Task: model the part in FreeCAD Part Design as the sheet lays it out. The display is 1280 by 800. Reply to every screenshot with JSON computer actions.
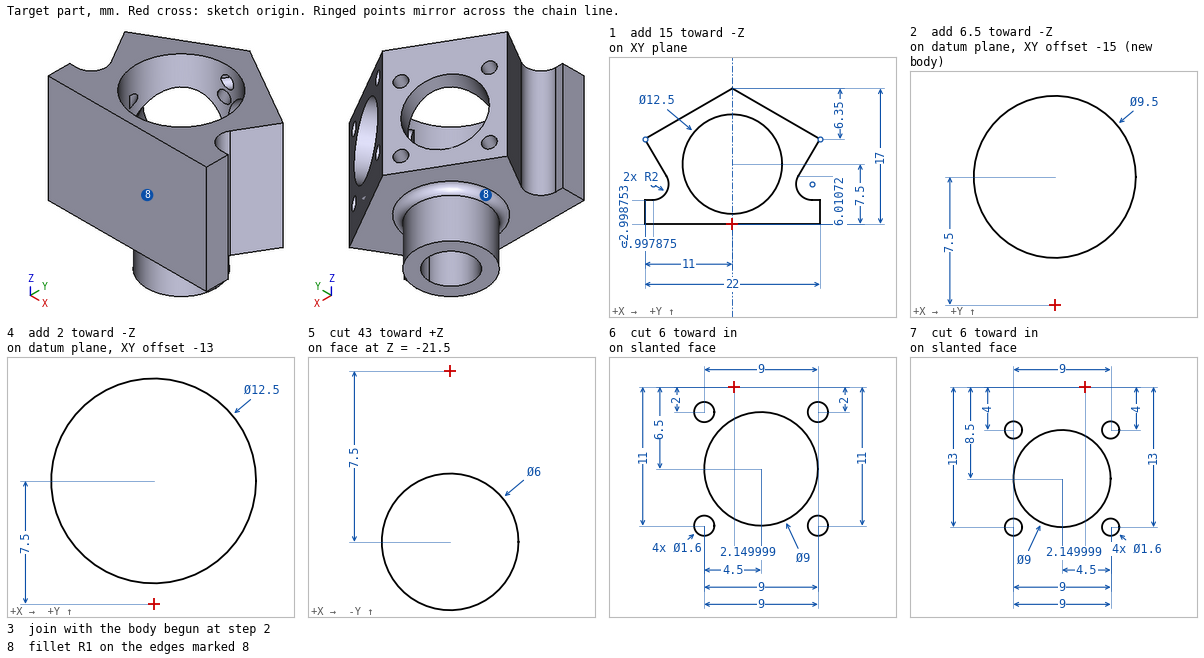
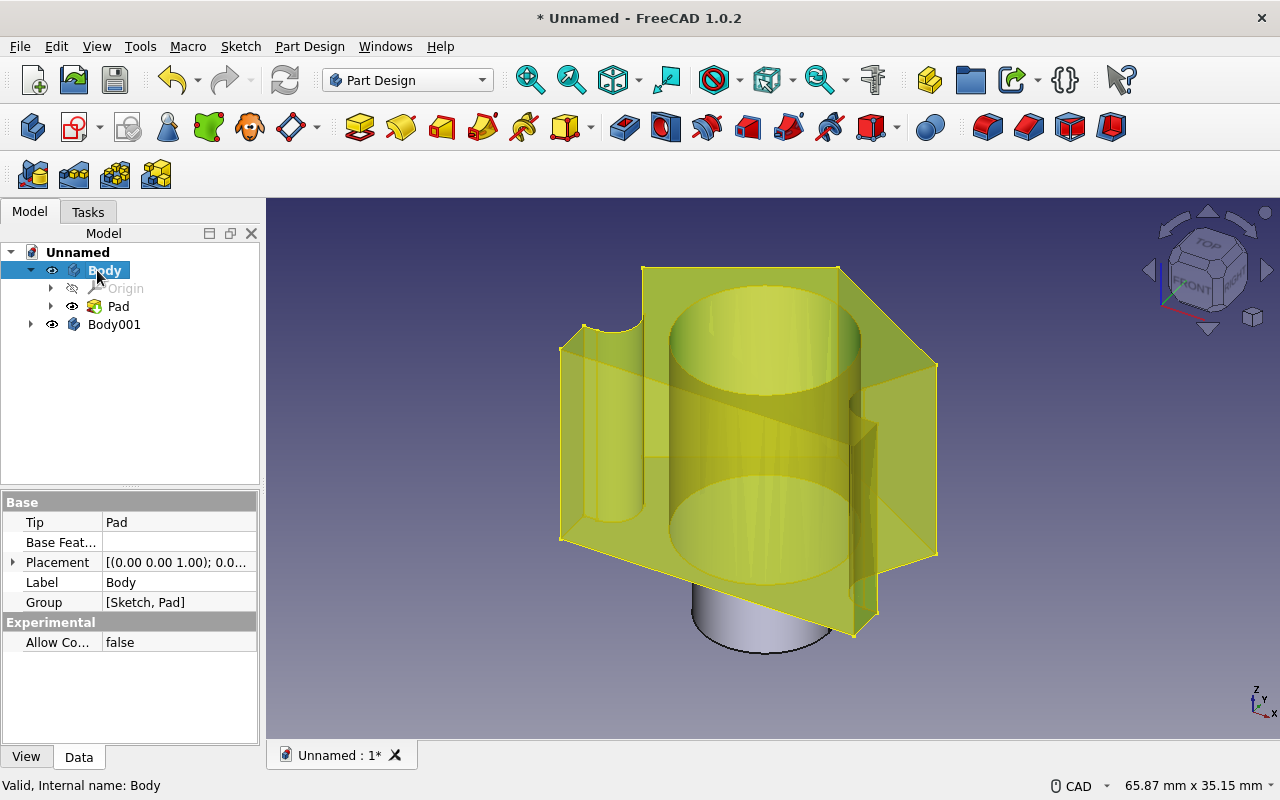
{"action": "left_click", "coordinate": [148, 642]}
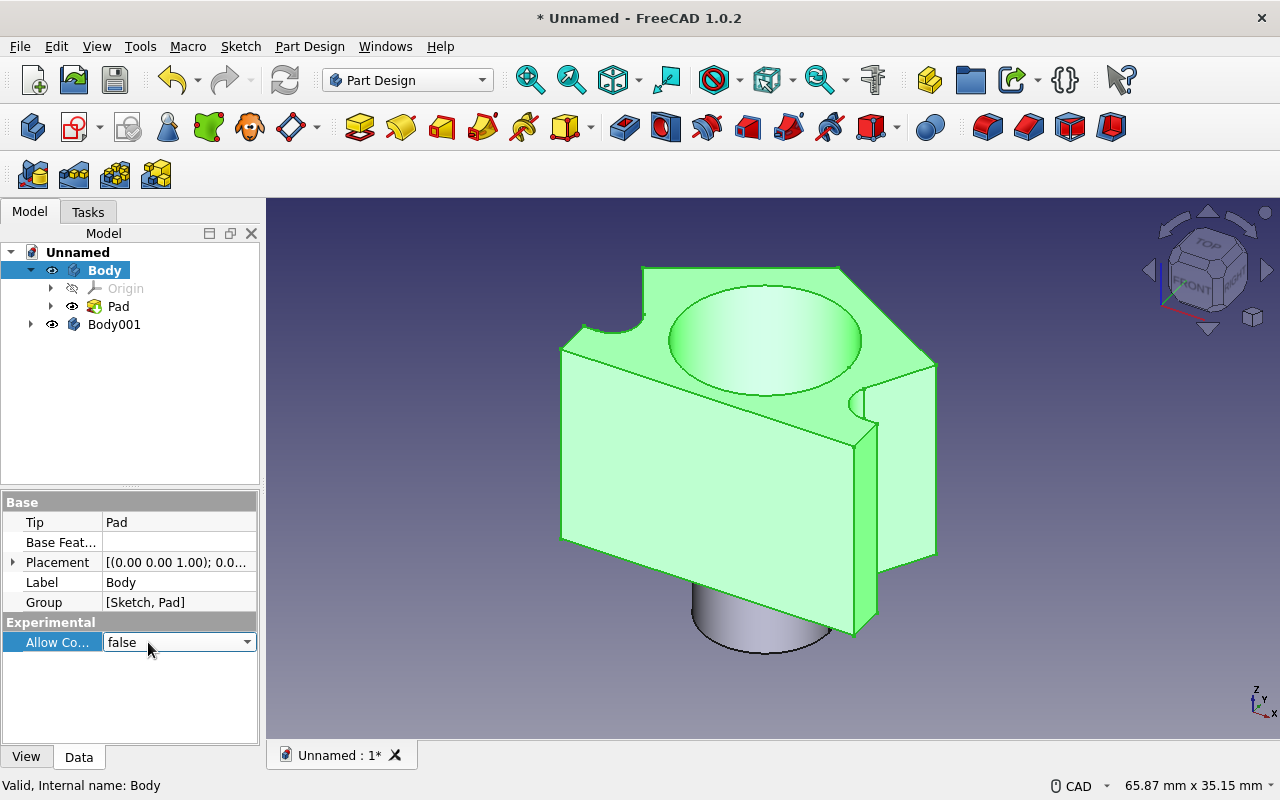
{"action": "left_click", "coordinate": [148, 642]}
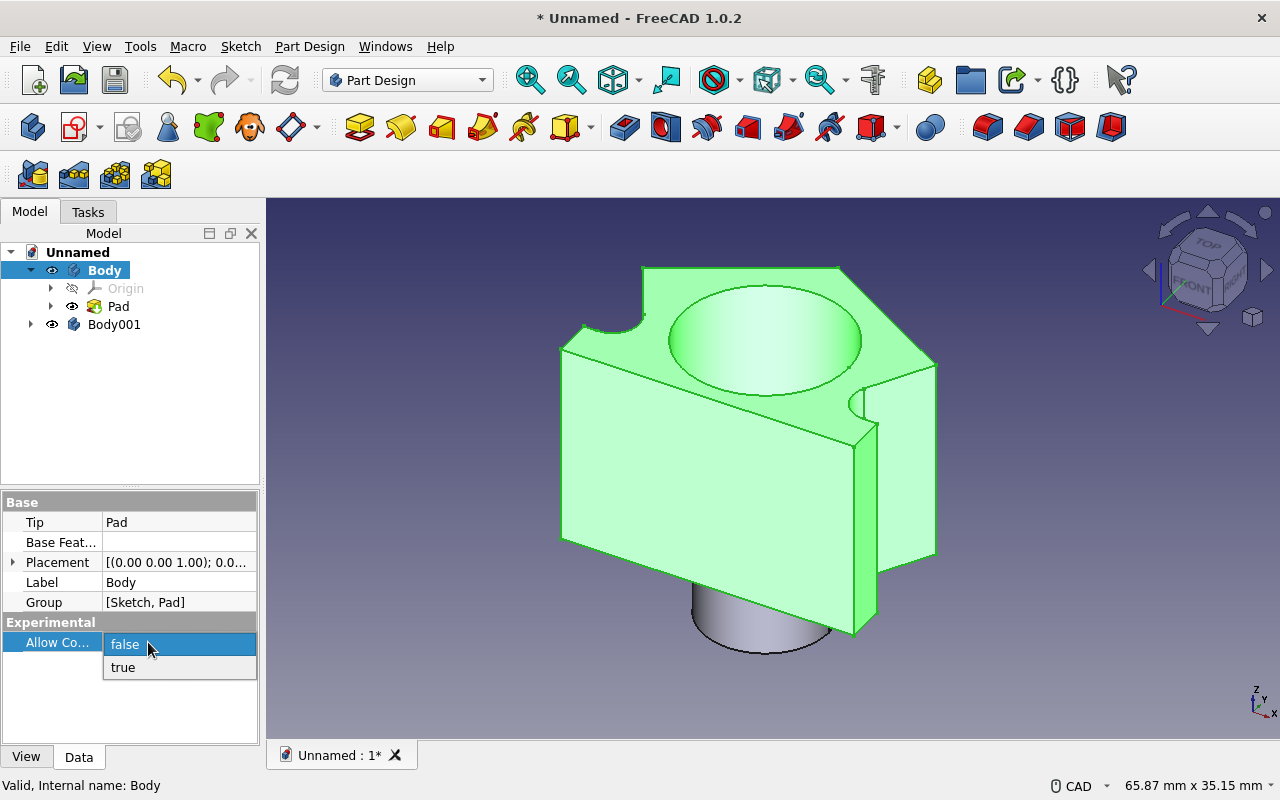
{"action": "left_click", "coordinate": [178, 668]}
{"action": "key", "text": "Return"}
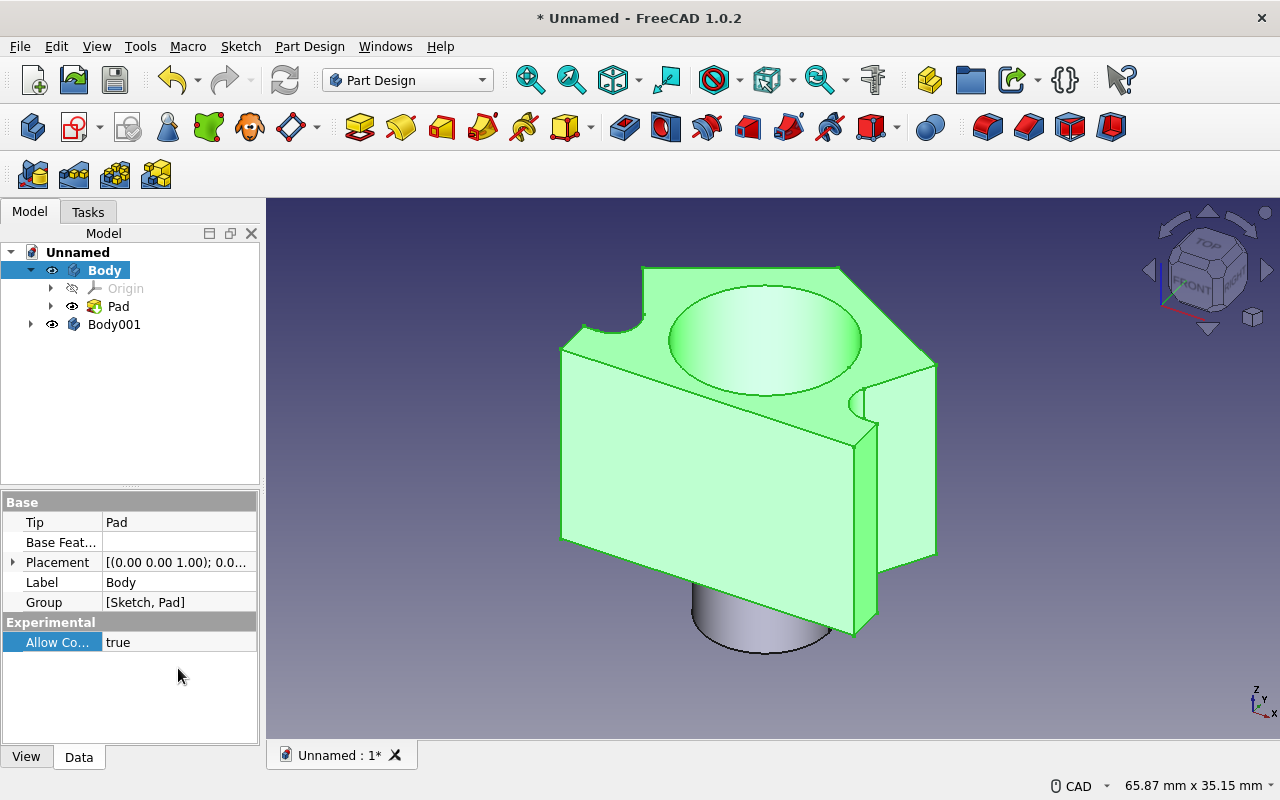
{"action": "left_click", "coordinate": [97, 324]}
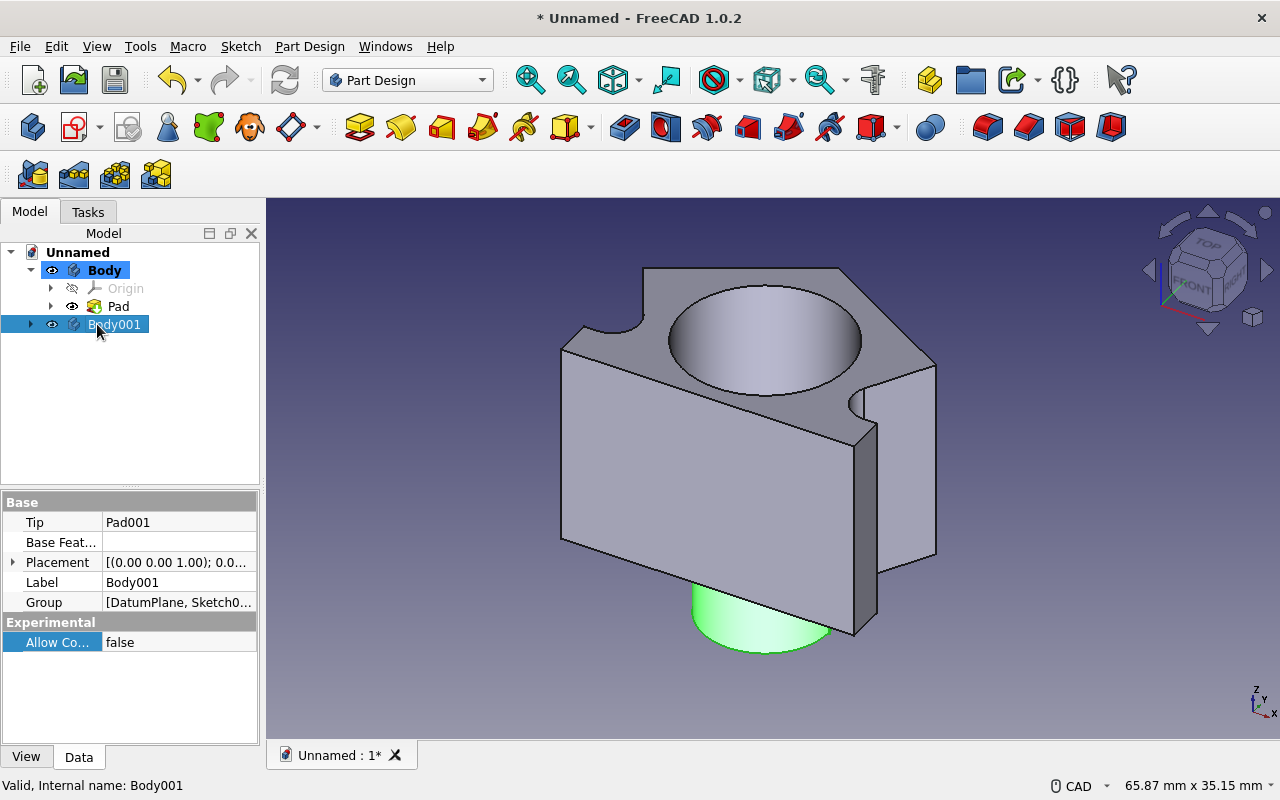
{"action": "left_click", "coordinate": [931, 128]}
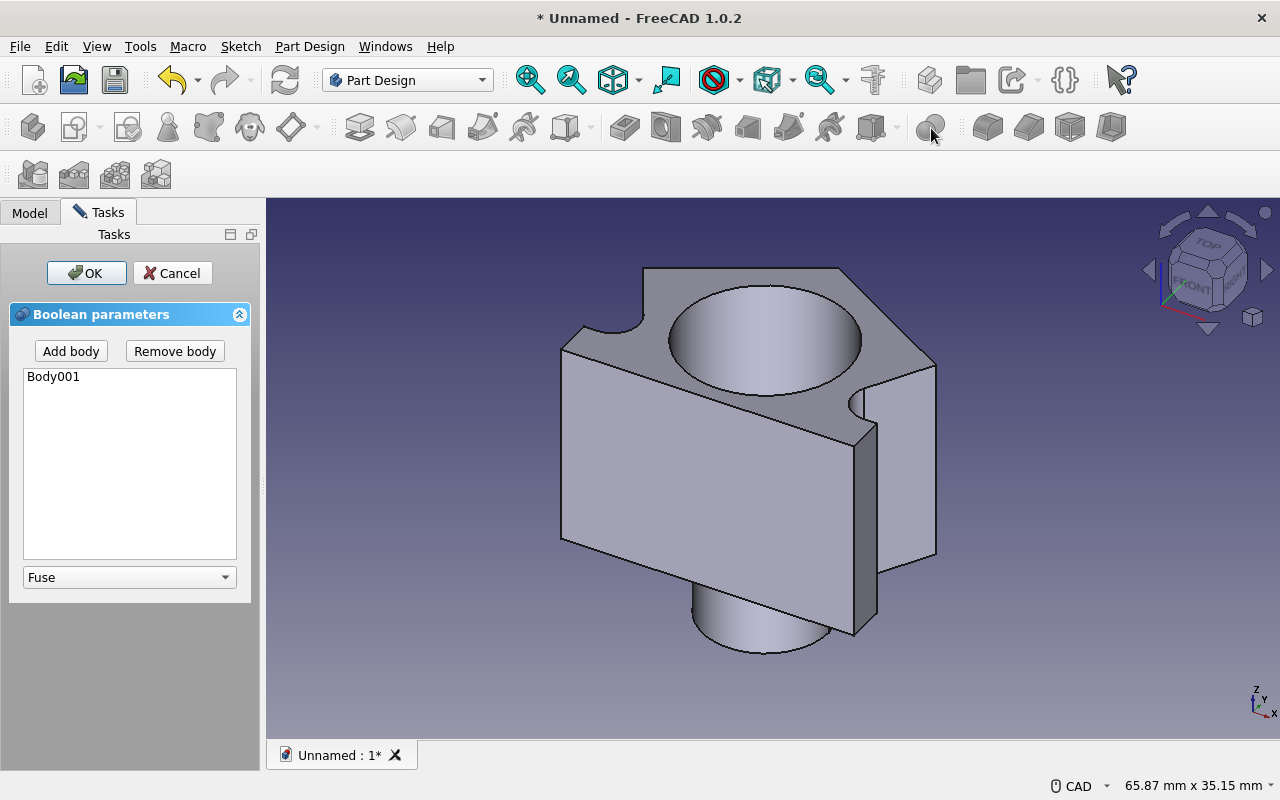
{"action": "left_click", "coordinate": [87, 273]}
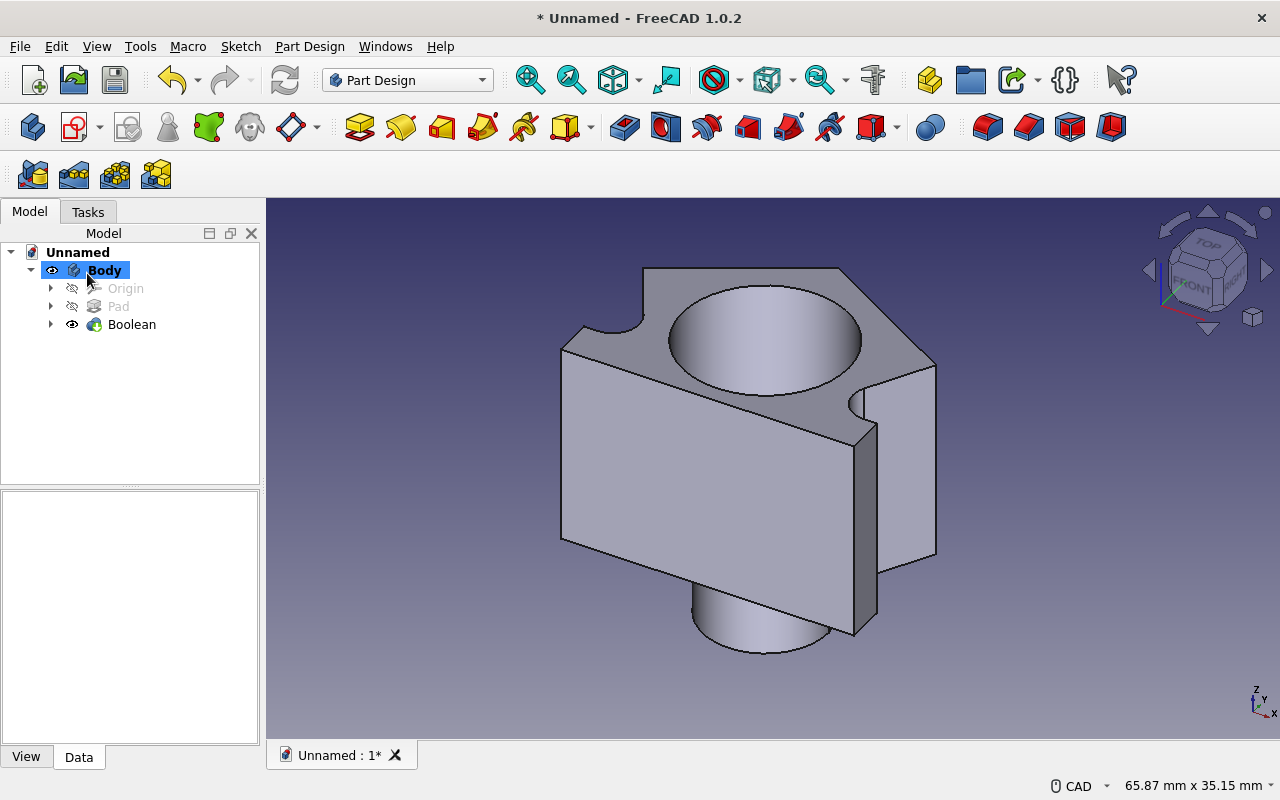
{"action": "left_click", "coordinate": [51, 288]}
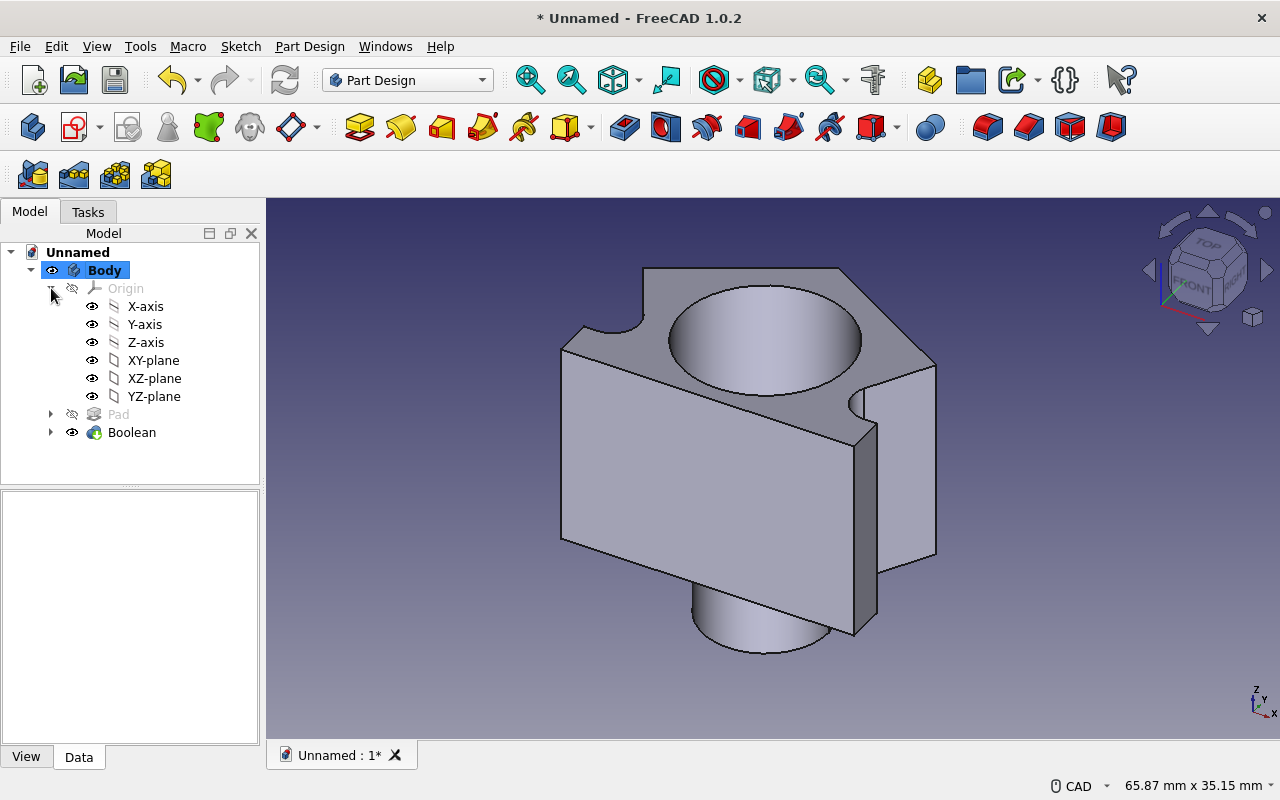
{"action": "left_click", "coordinate": [137, 360]}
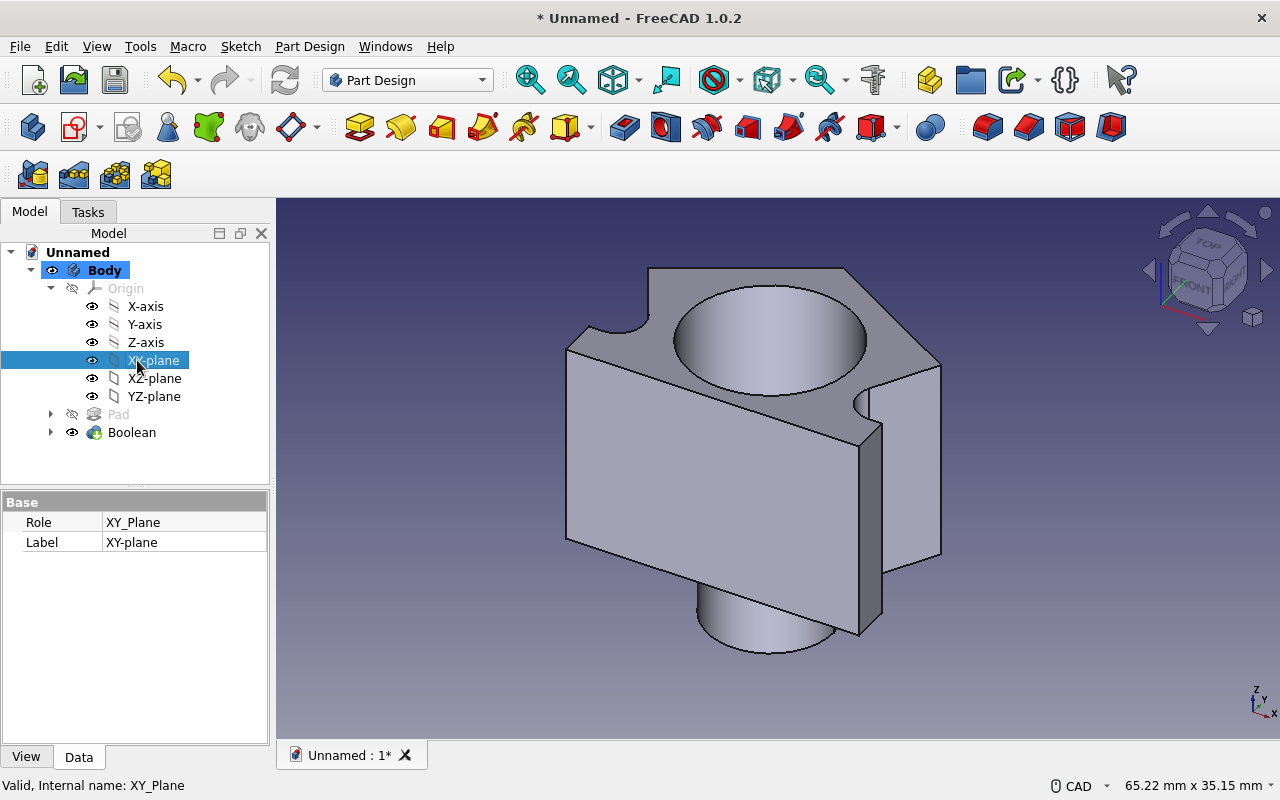
{"action": "left_click", "coordinate": [290, 128]}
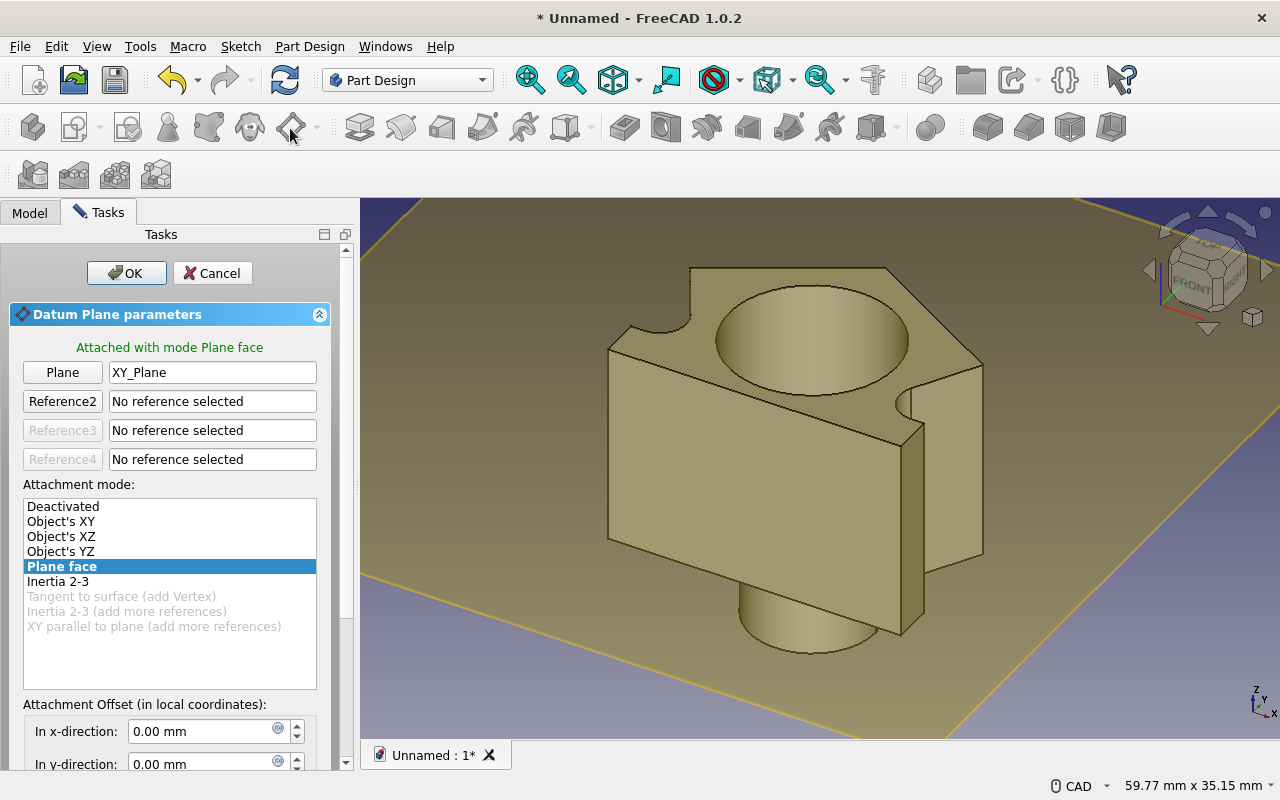
{"action": "scroll", "coordinate": [346, 507], "scroll_direction": "down", "scroll_amount": 2}